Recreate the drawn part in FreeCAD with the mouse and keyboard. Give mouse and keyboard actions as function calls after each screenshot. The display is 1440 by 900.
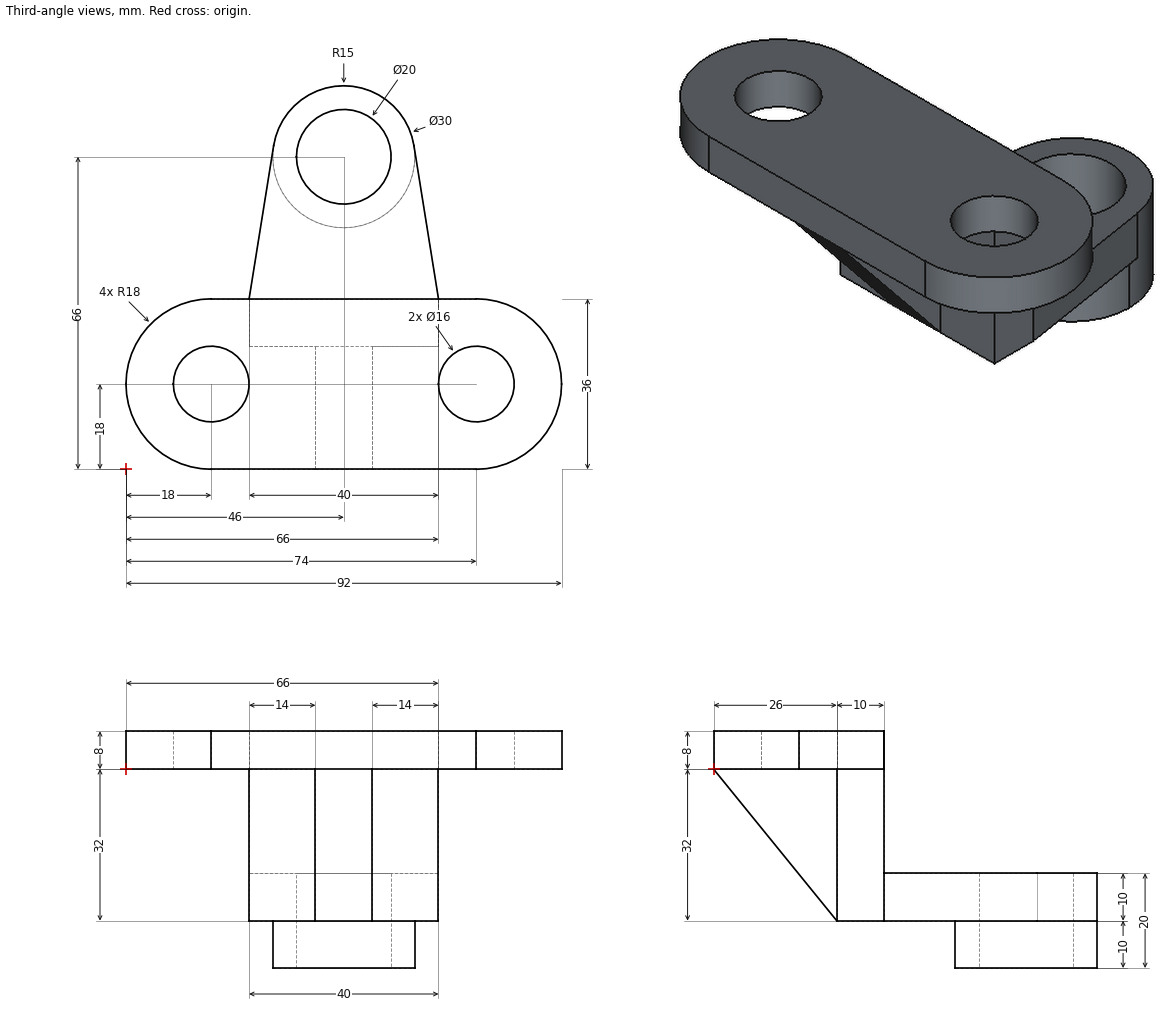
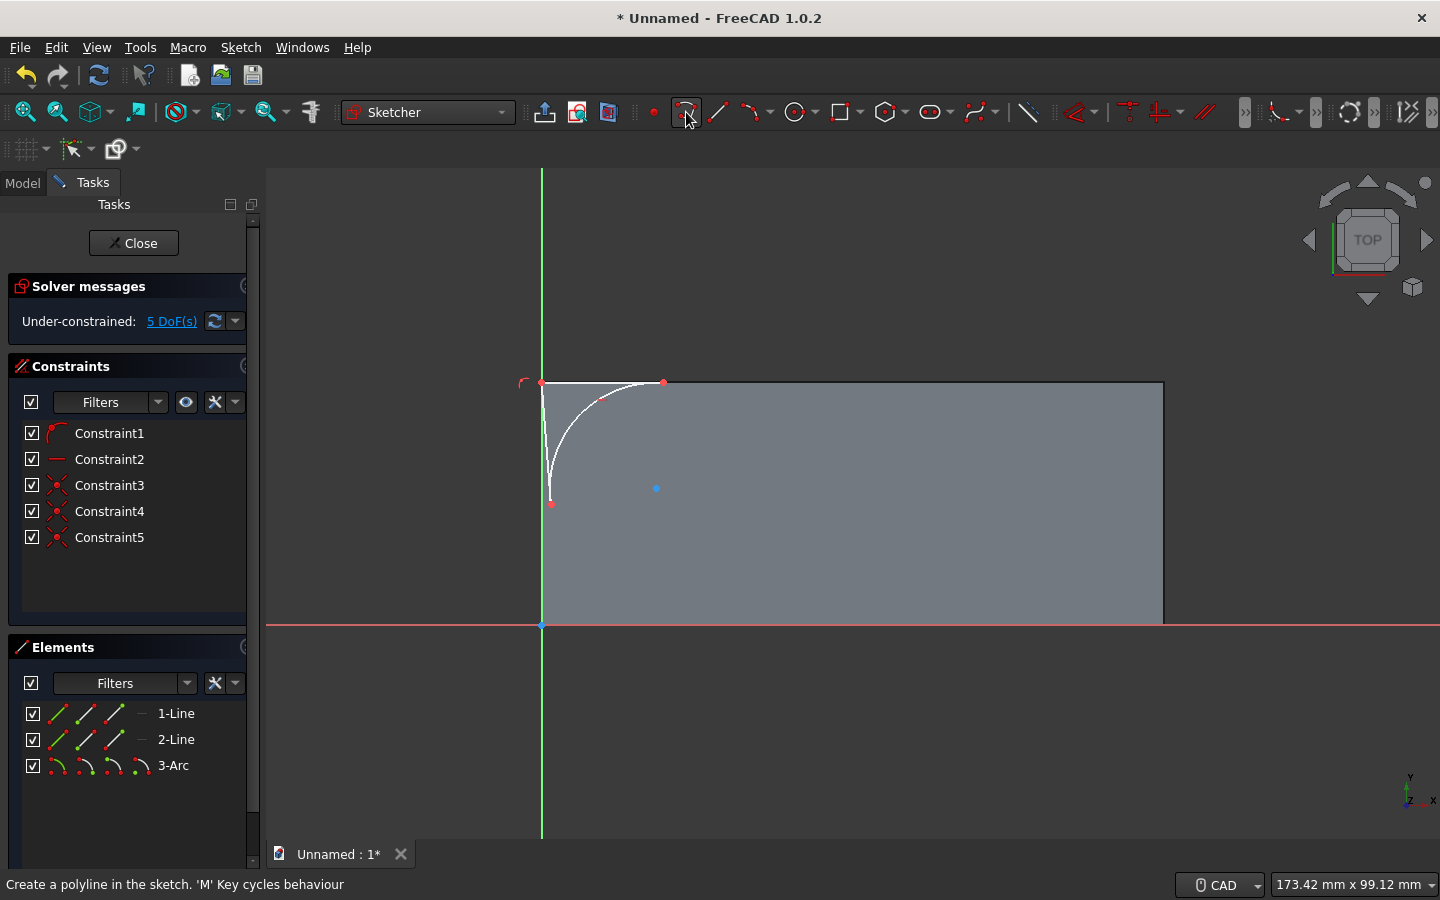
click(551, 505)
click(551, 625)
click(663, 616)
right_click(663, 616)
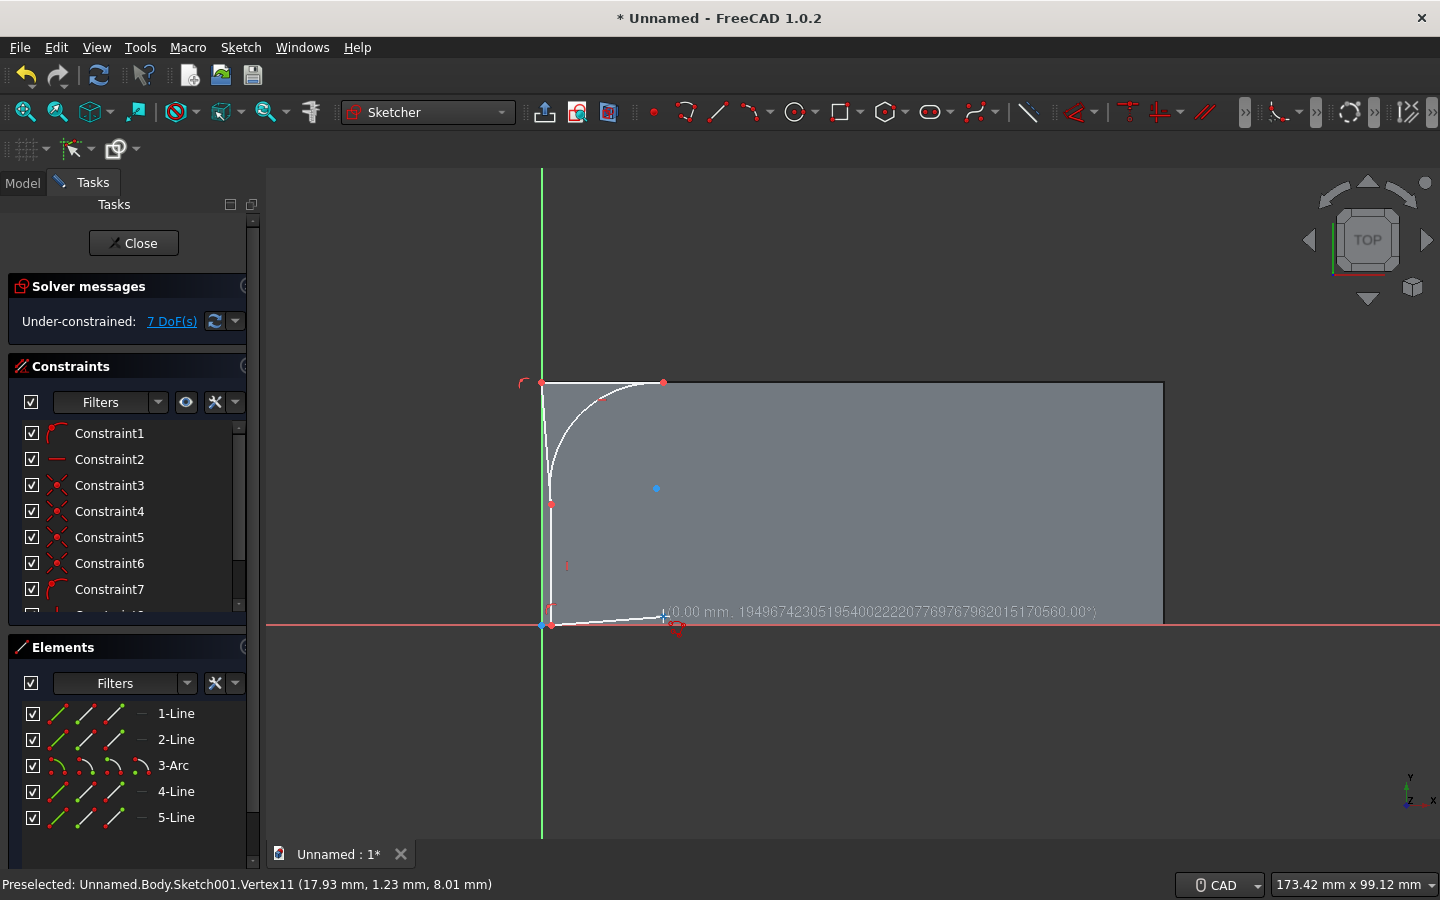
click(750, 112)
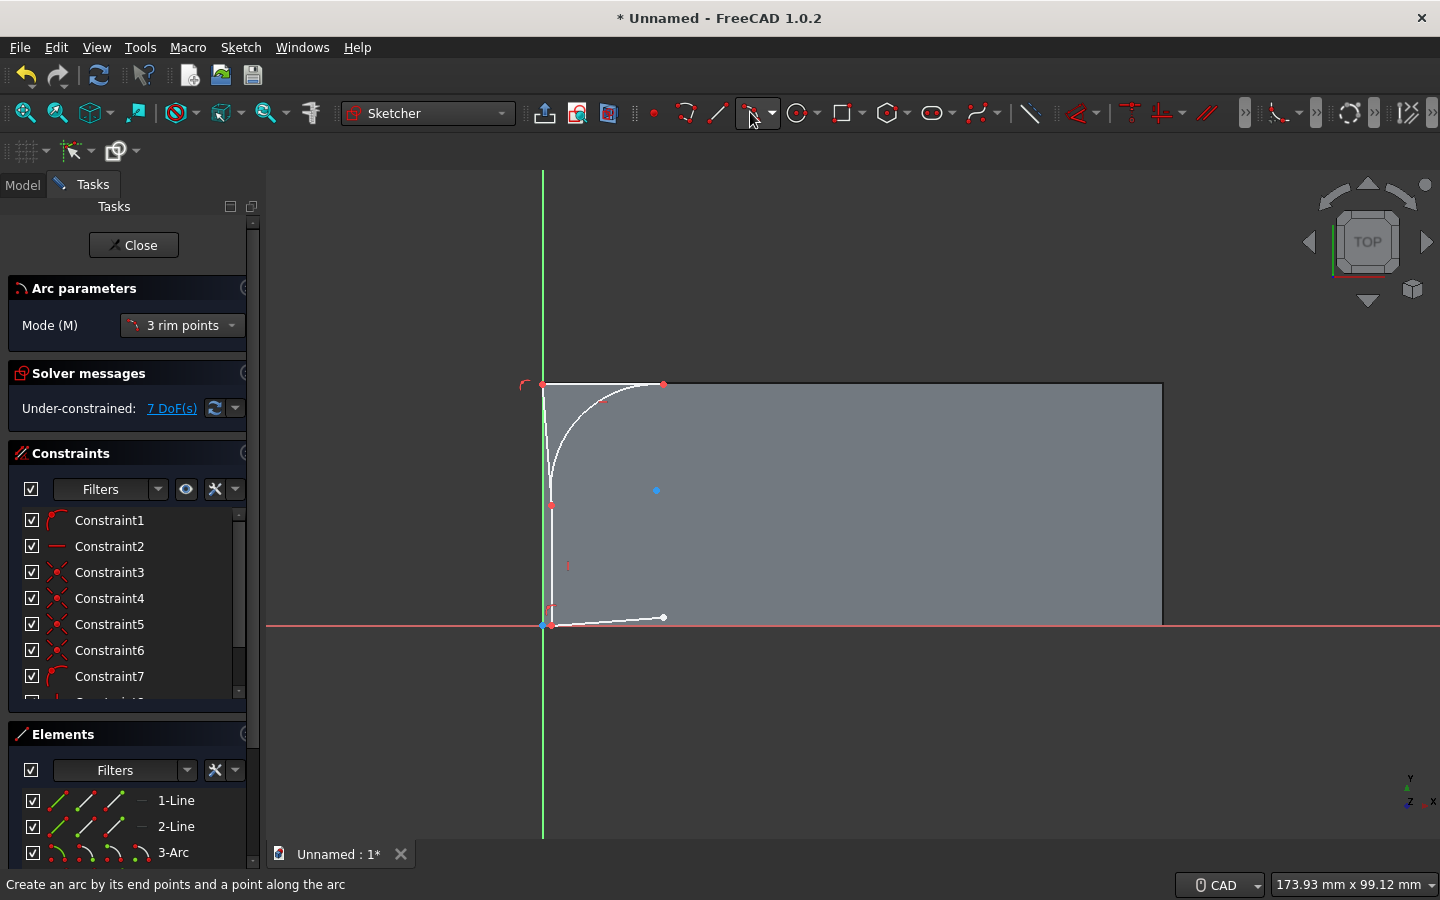
click(664, 618)
click(552, 506)
click(578, 590)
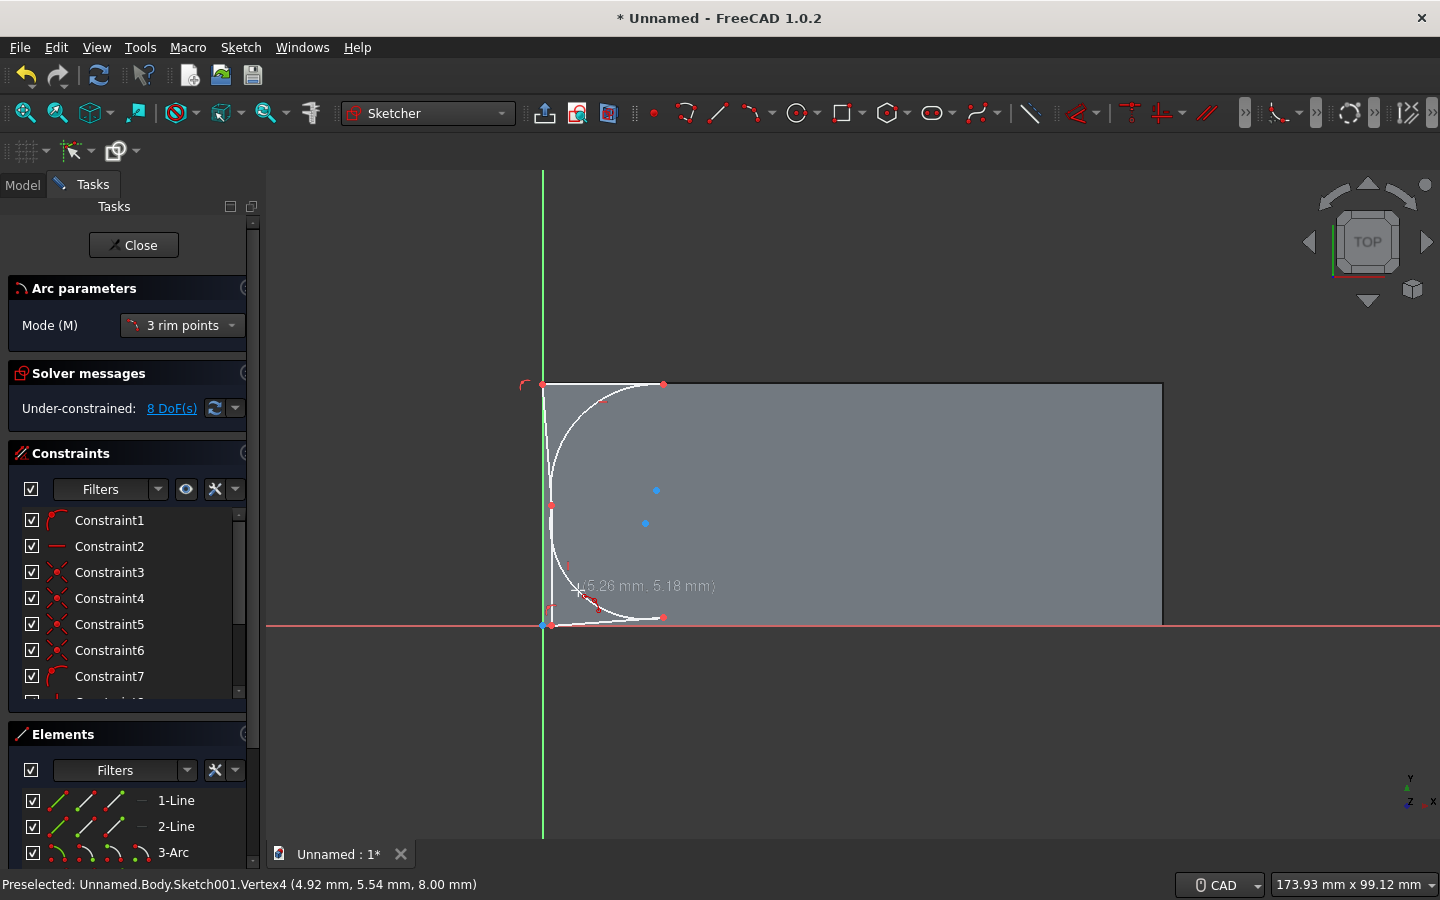
click(686, 114)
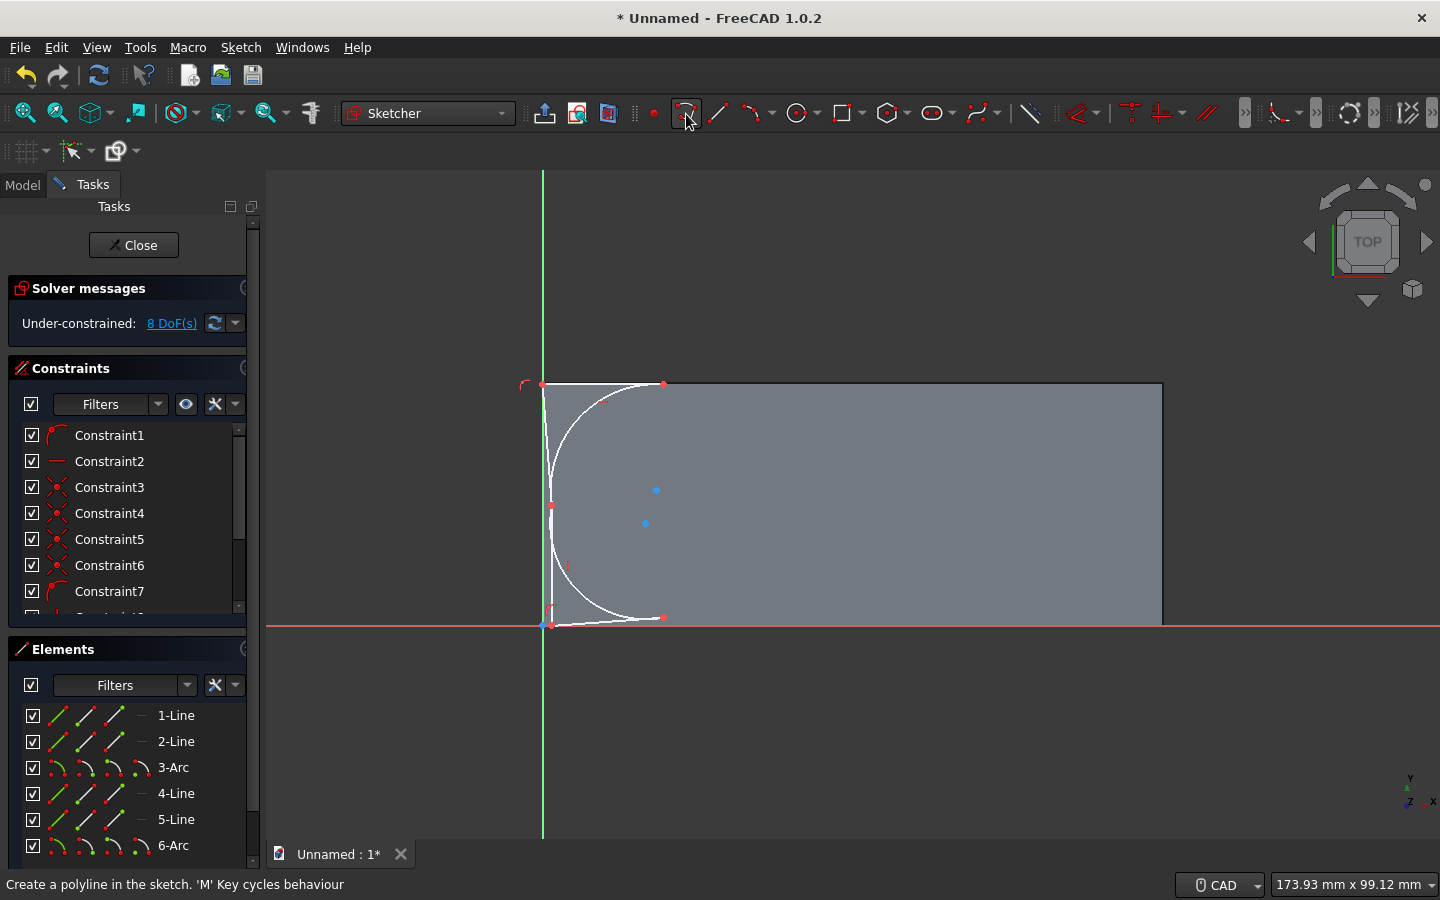
click(1042, 626)
click(1163, 617)
click(1163, 505)
right_click(1163, 505)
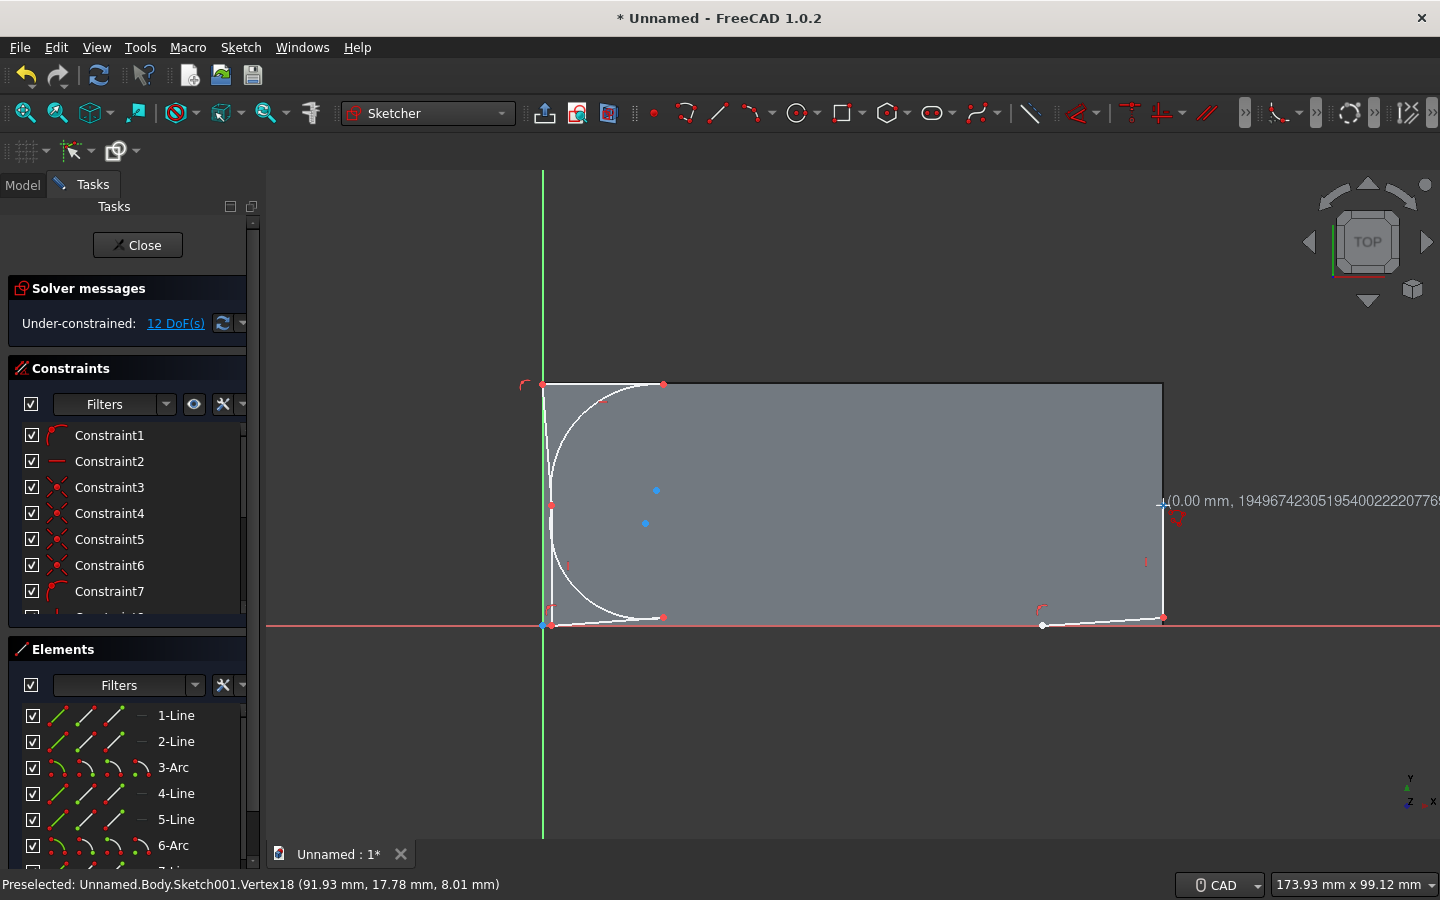
click(752, 114)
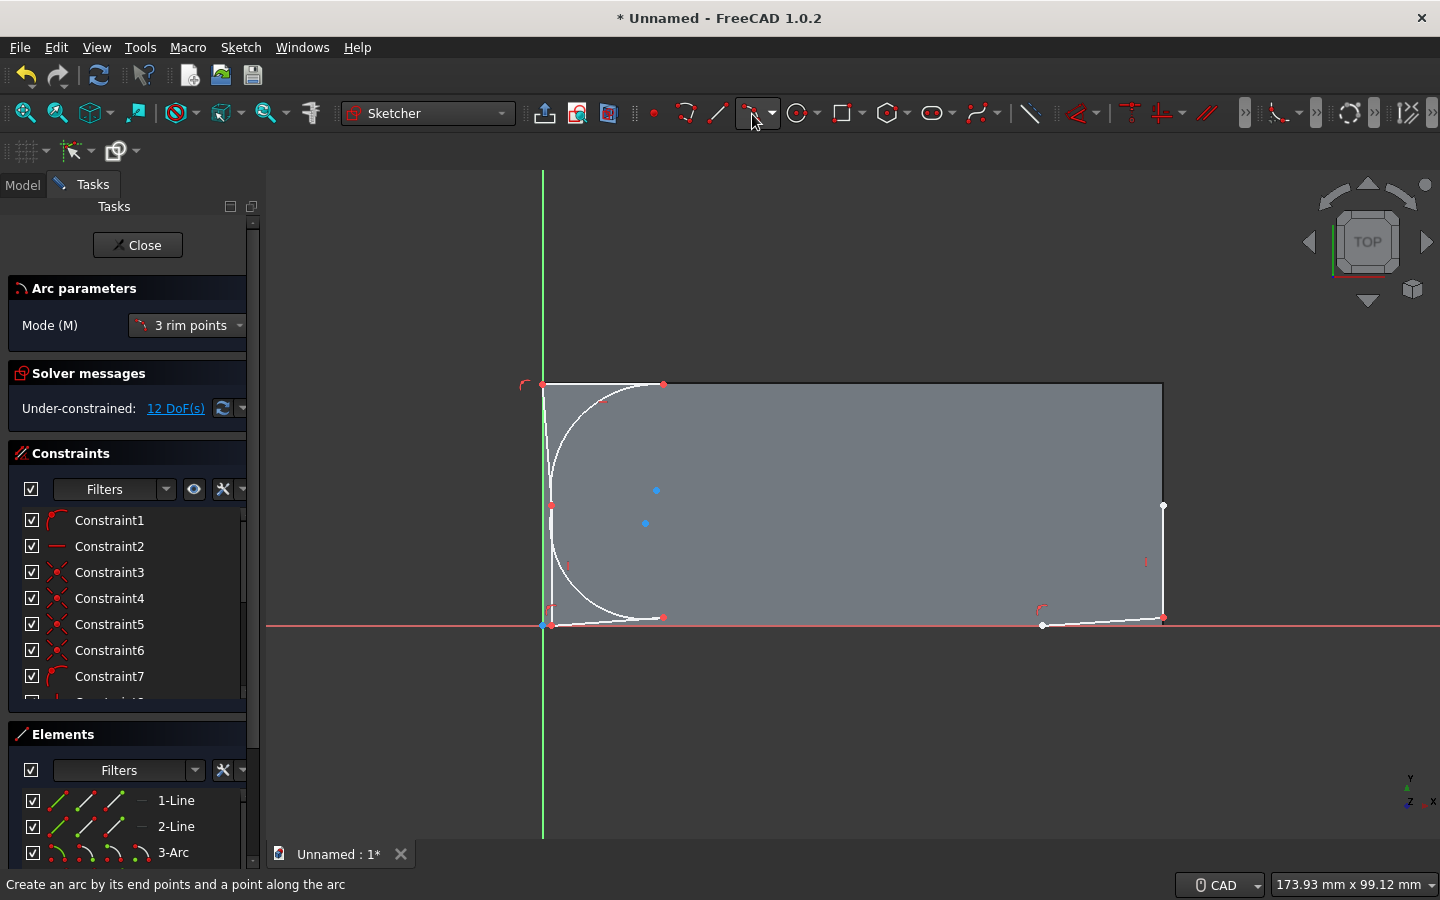
click(1163, 506)
click(1042, 626)
click(1128, 590)